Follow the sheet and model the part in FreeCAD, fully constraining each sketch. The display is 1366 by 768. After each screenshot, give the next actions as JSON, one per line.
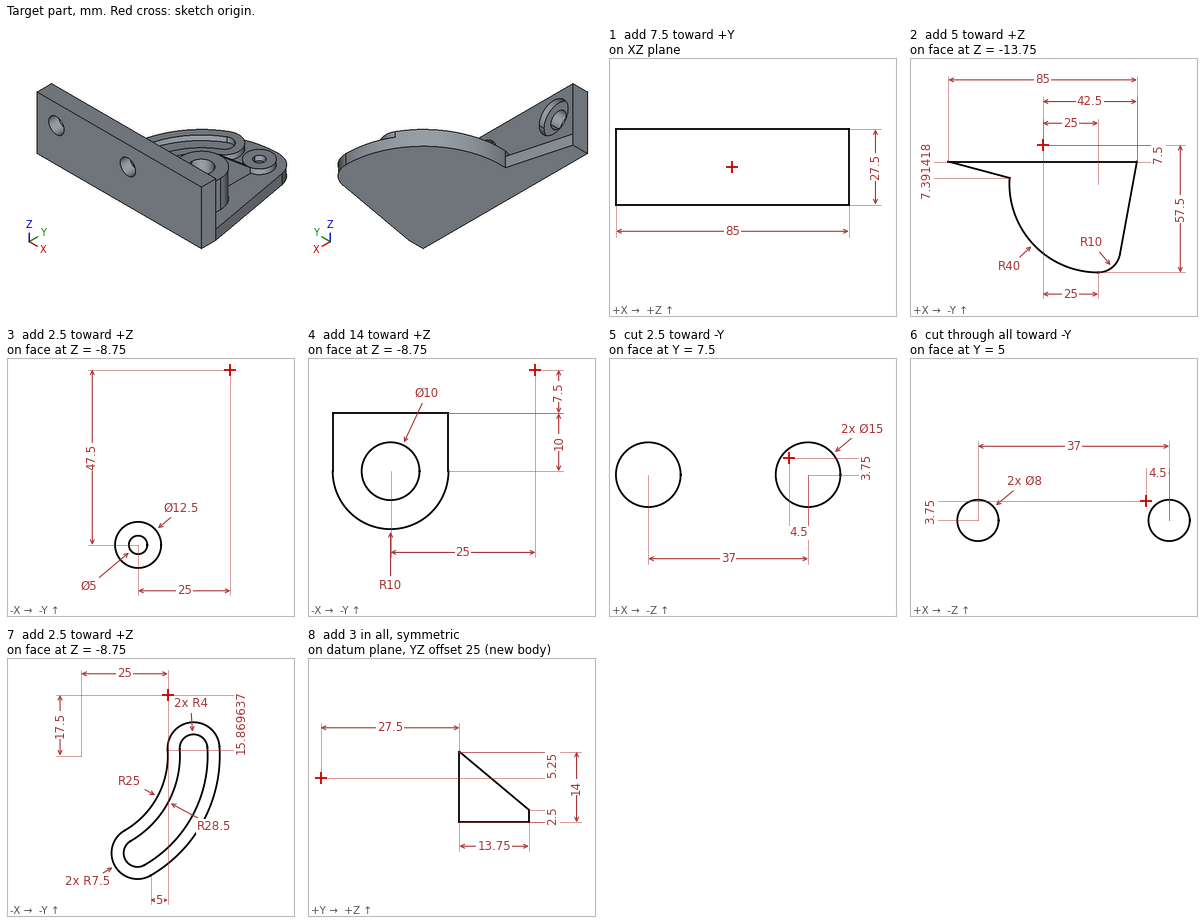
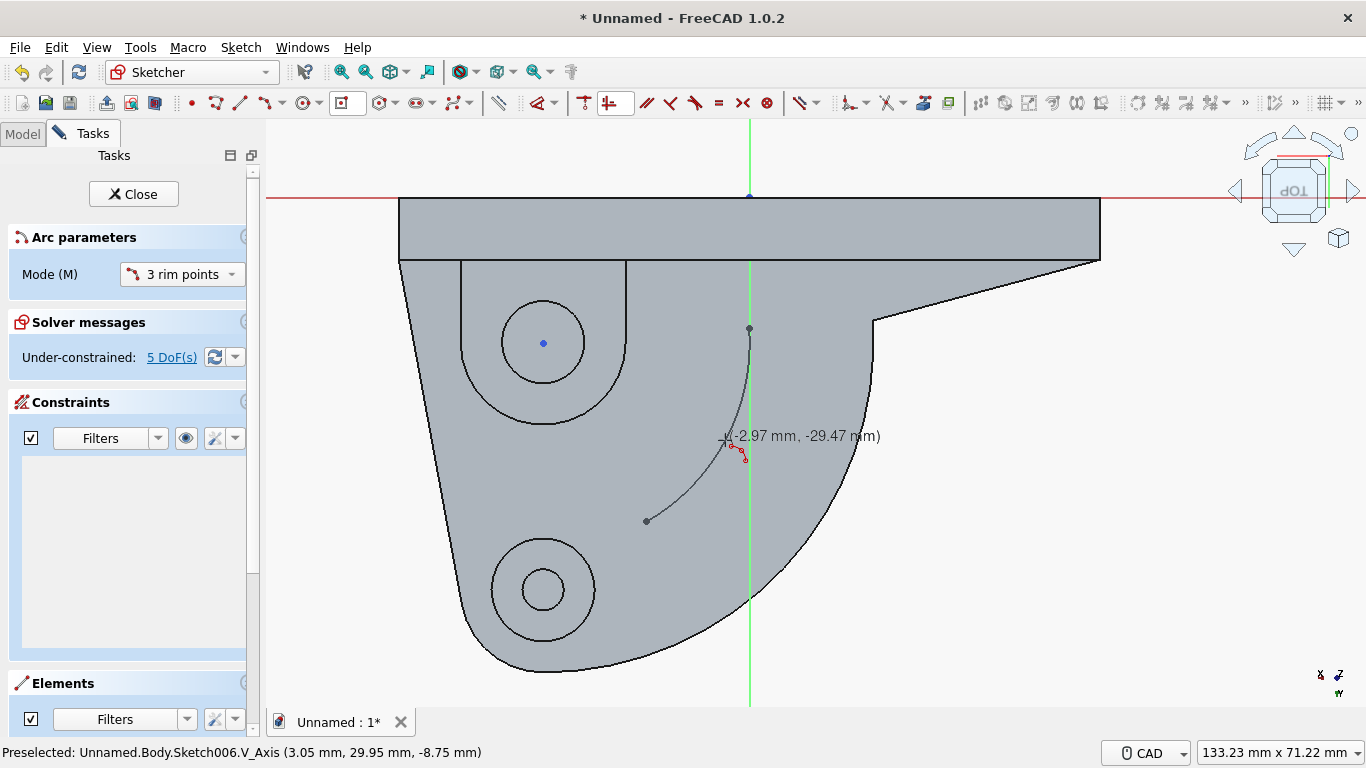
{"action": "left_click", "coordinate": [646, 522]}
{"action": "left_click", "coordinate": [708, 628]}
{"action": "left_click", "coordinate": [624, 606]}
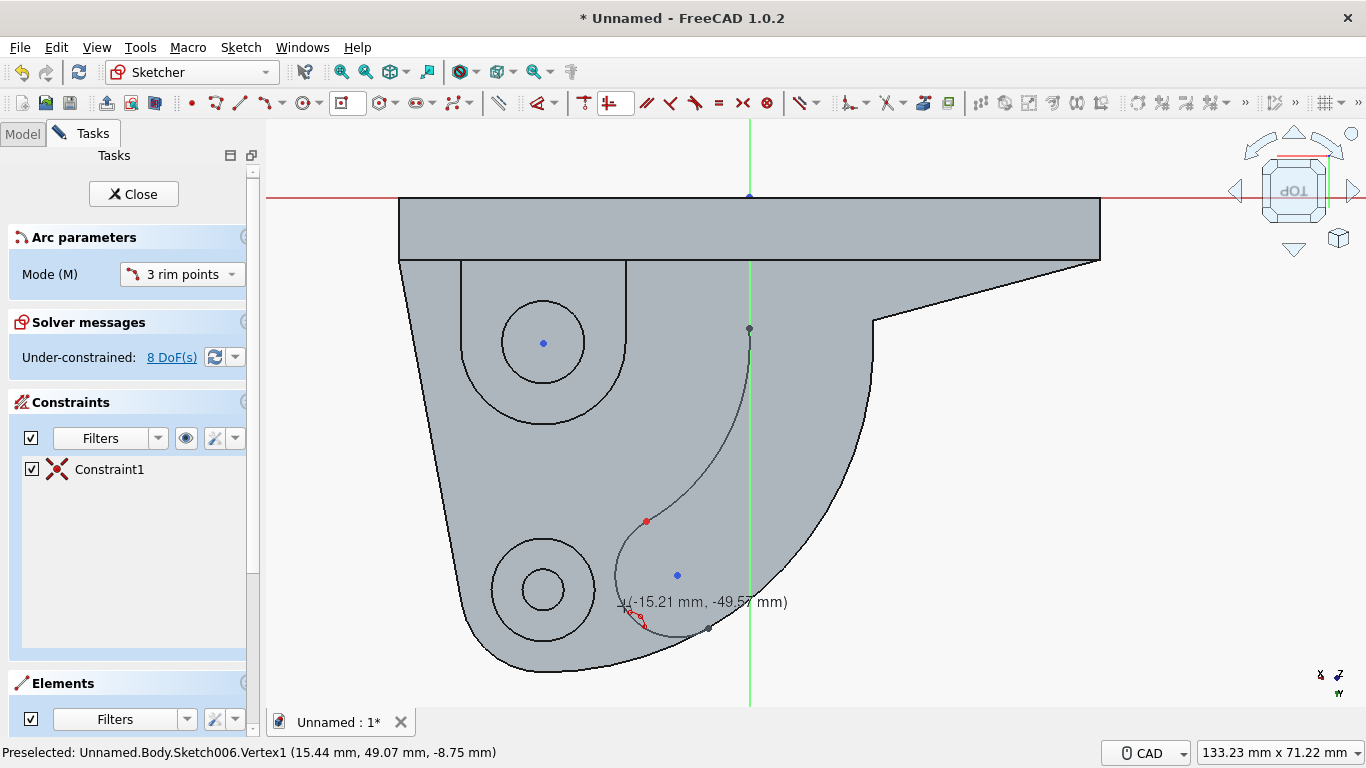
{"action": "left_click", "coordinate": [708, 629]}
{"action": "left_click", "coordinate": [873, 321]}
{"action": "left_click", "coordinate": [834, 498]}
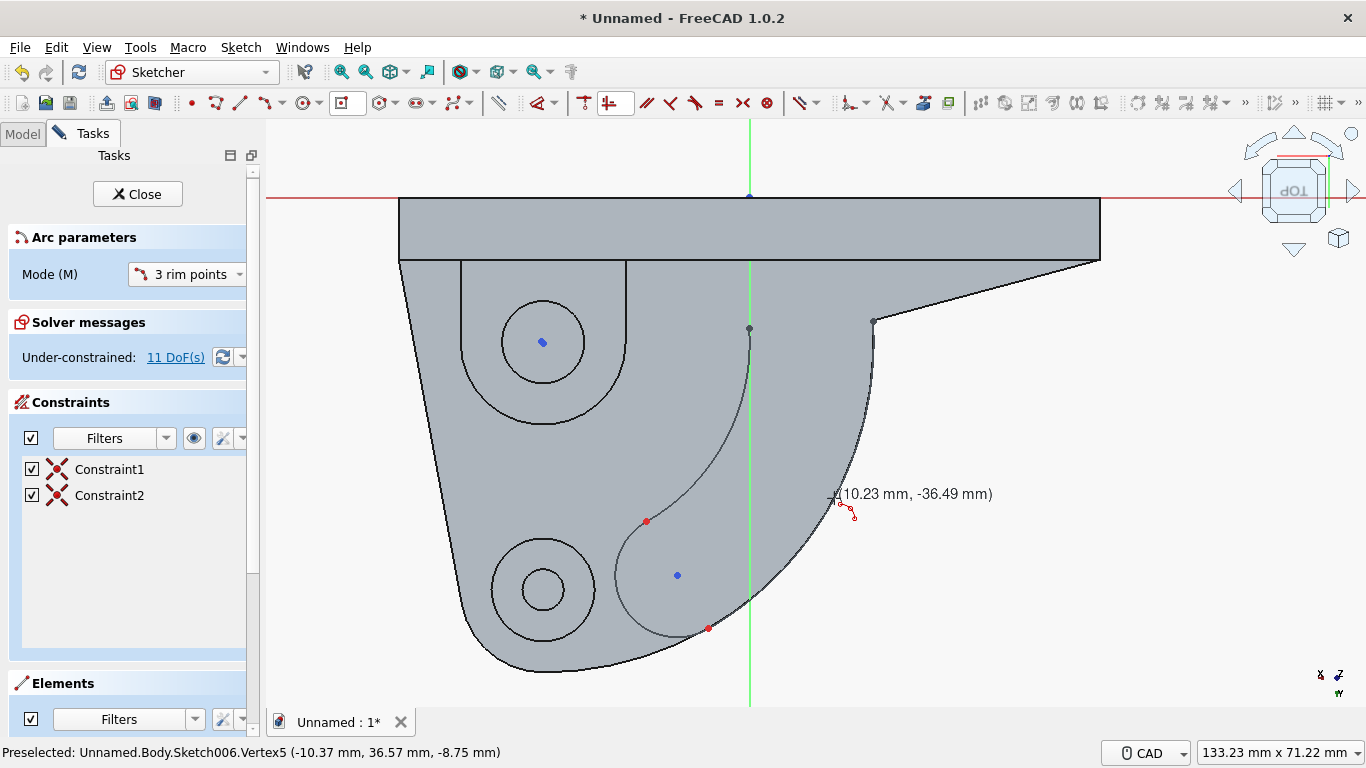
{"action": "left_click", "coordinate": [873, 322]}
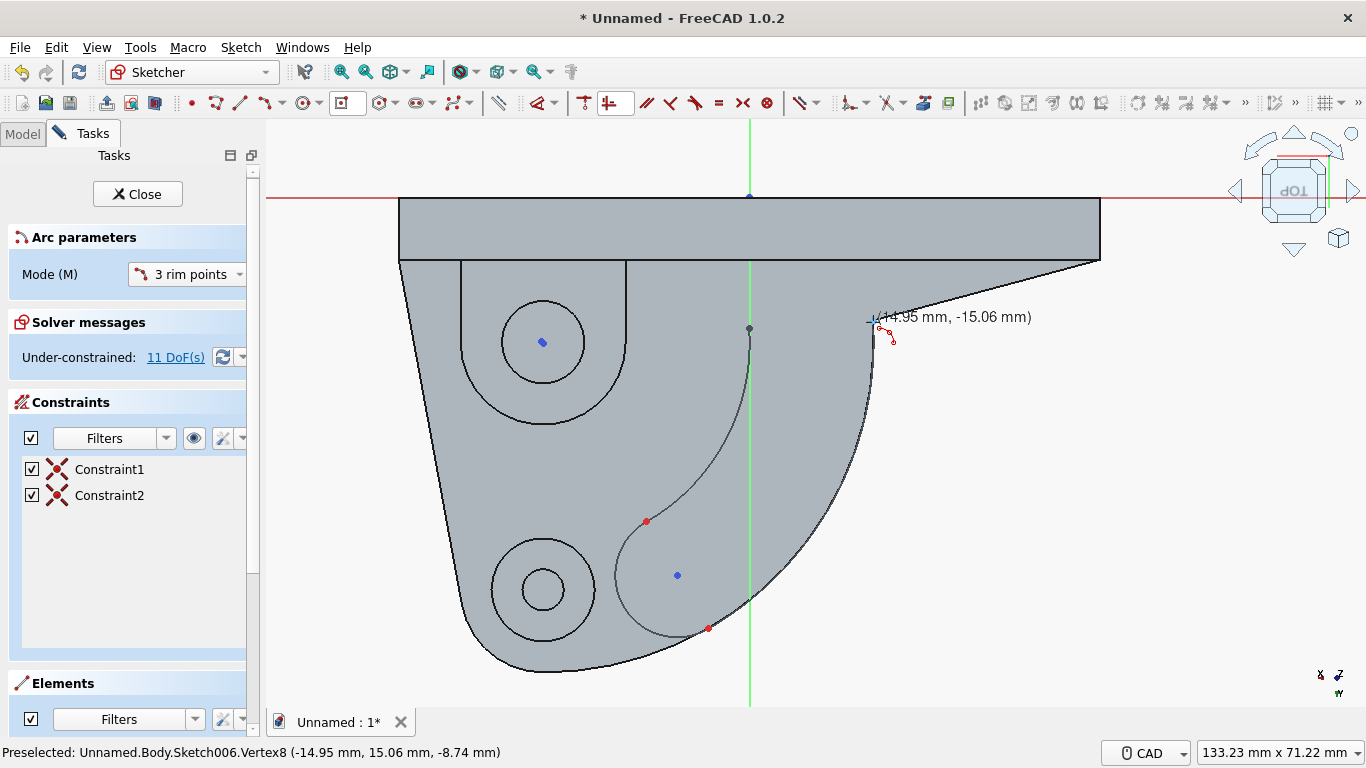
{"action": "scroll", "coordinate": [749, 329], "scroll_direction": "up", "scroll_amount": 18}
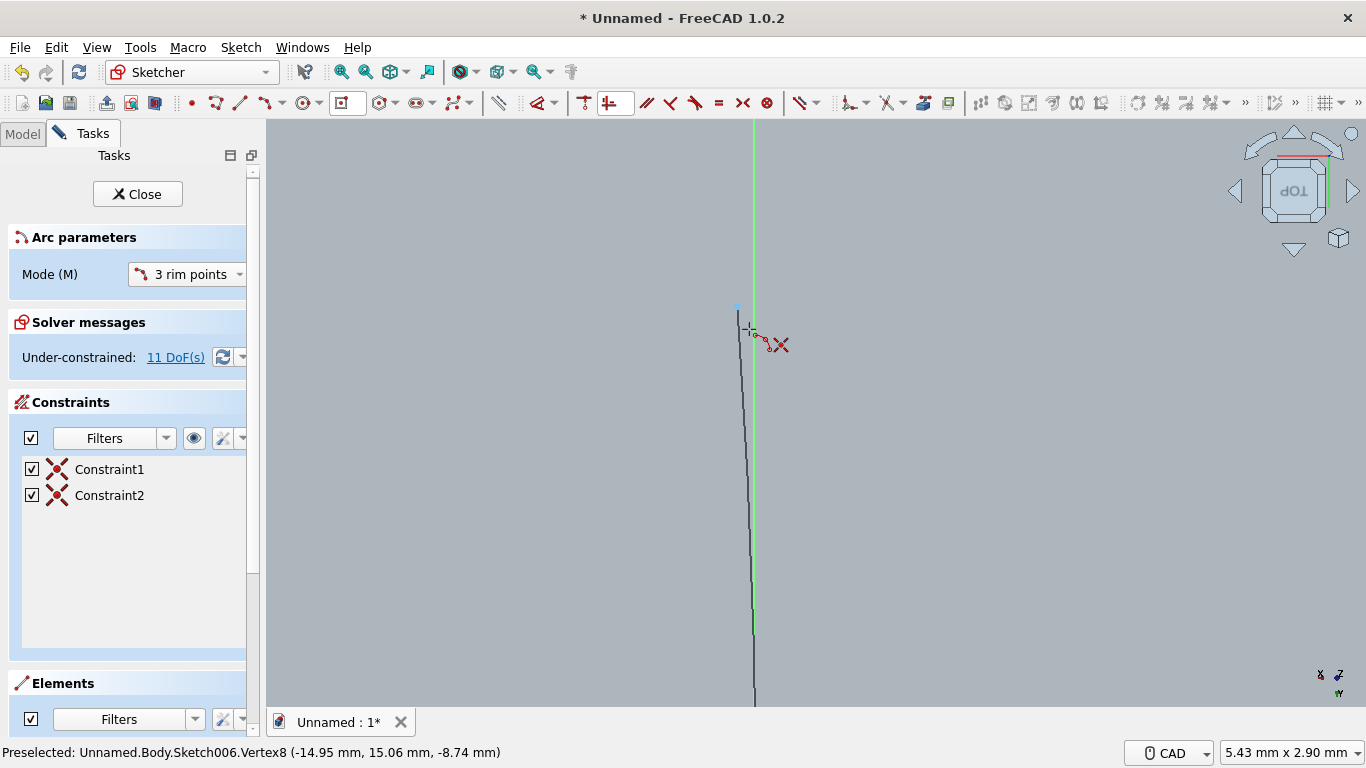
{"action": "left_click", "coordinate": [737, 307]}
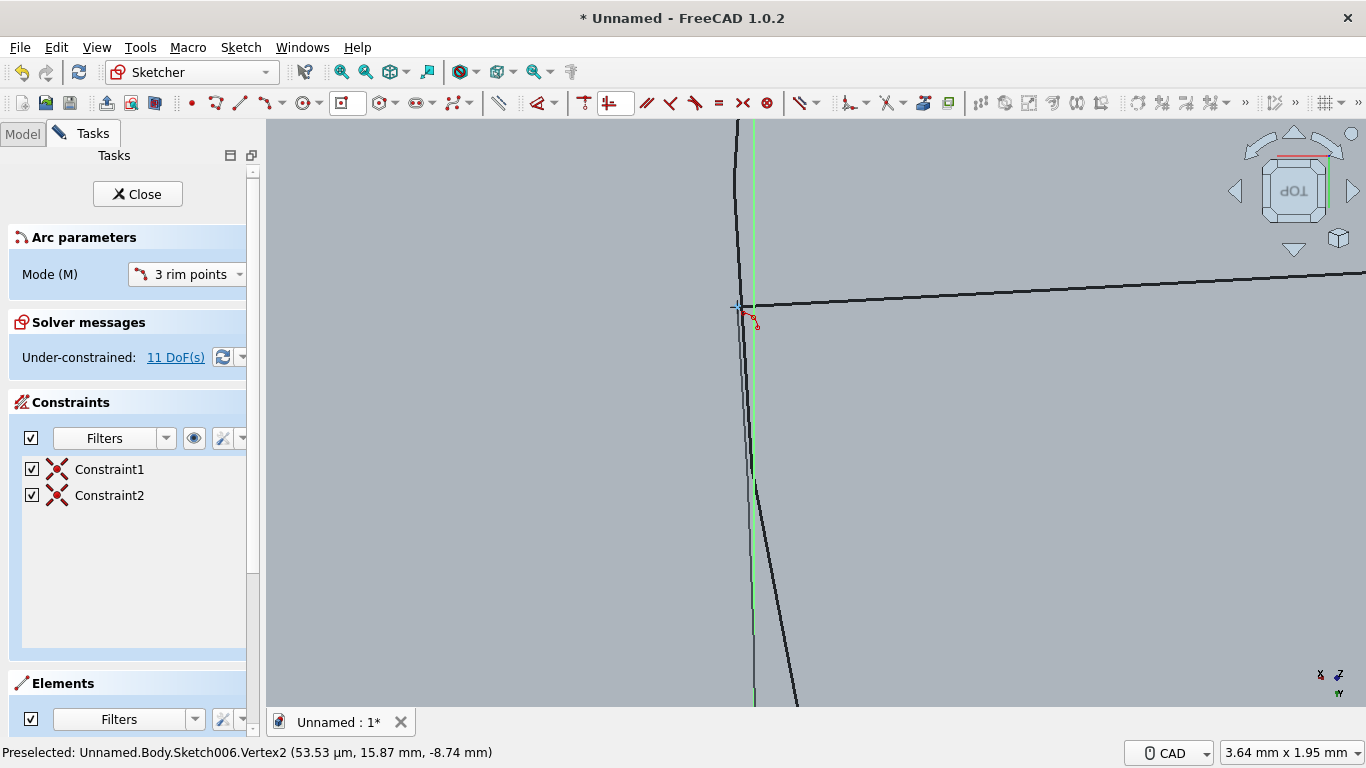
{"action": "scroll", "coordinate": [749, 329], "scroll_direction": "down", "scroll_amount": 18}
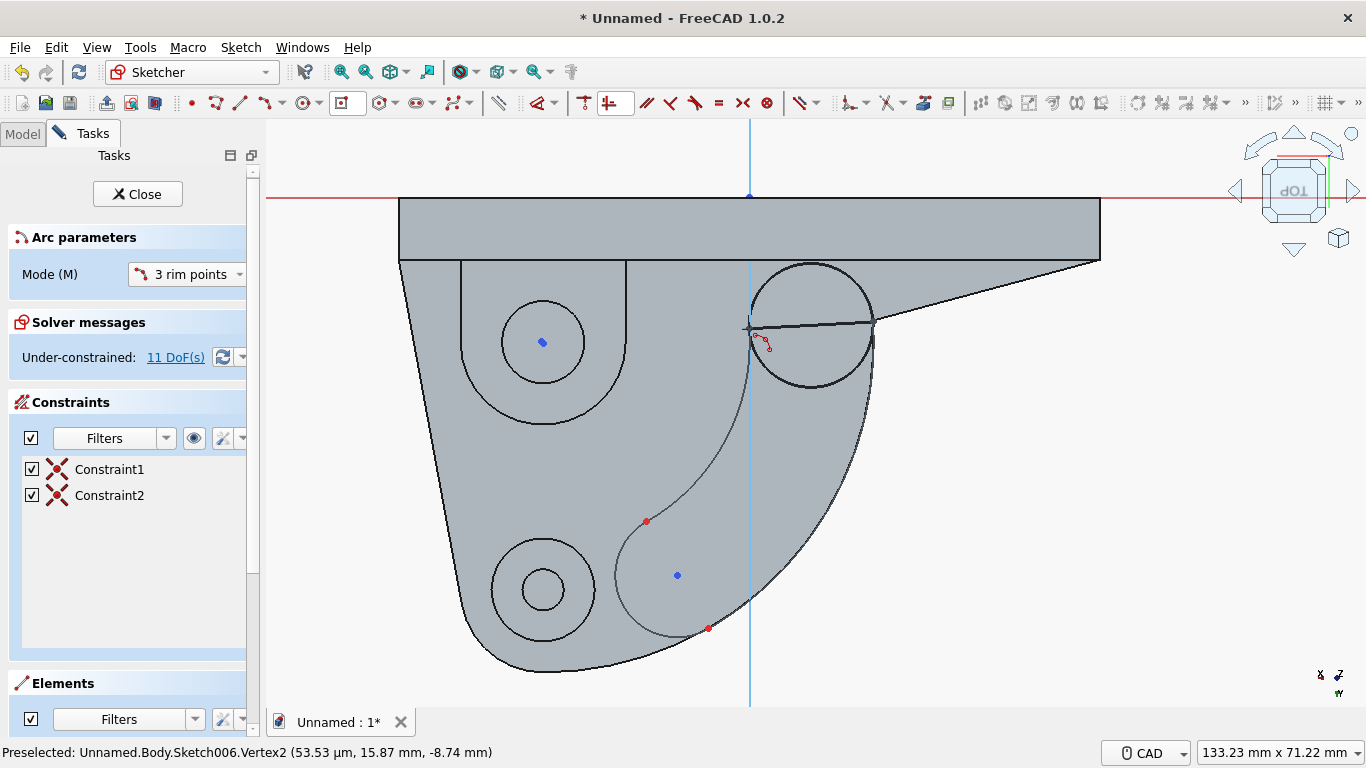
{"action": "left_click", "coordinate": [807, 263]}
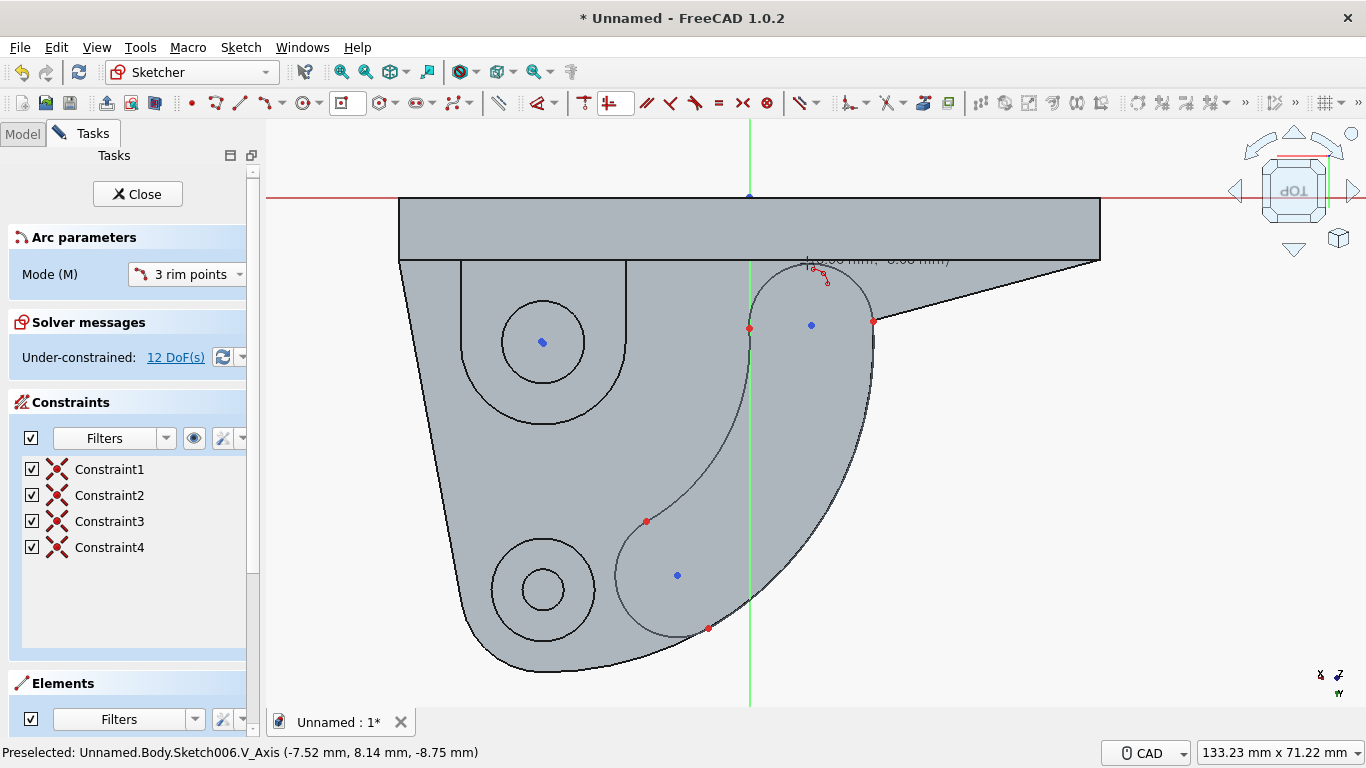
{"action": "left_click", "coordinate": [778, 327]}
{"action": "left_click", "coordinate": [844, 323]}
{"action": "left_click", "coordinate": [809, 292]}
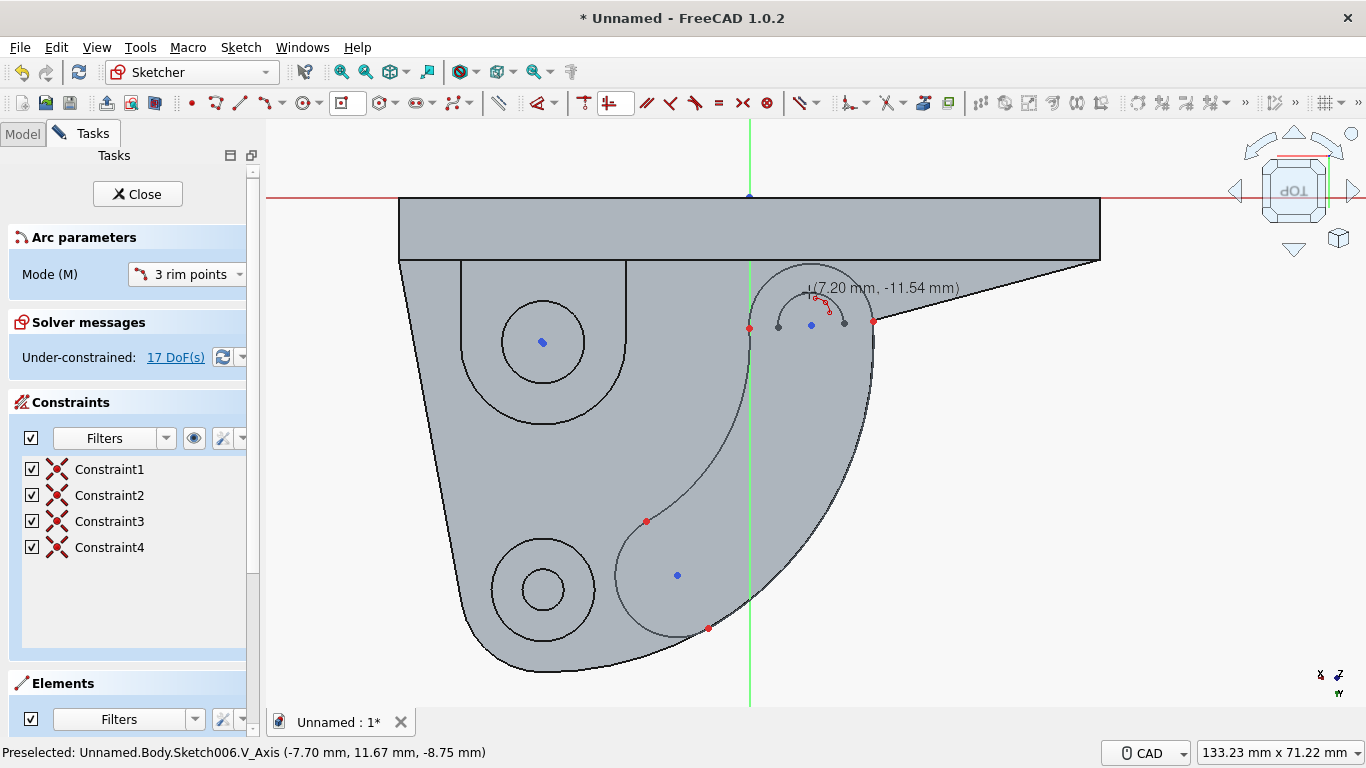
{"action": "left_click", "coordinate": [844, 324]}
{"action": "left_click", "coordinate": [694, 603]}
{"action": "left_click", "coordinate": [809, 484]}